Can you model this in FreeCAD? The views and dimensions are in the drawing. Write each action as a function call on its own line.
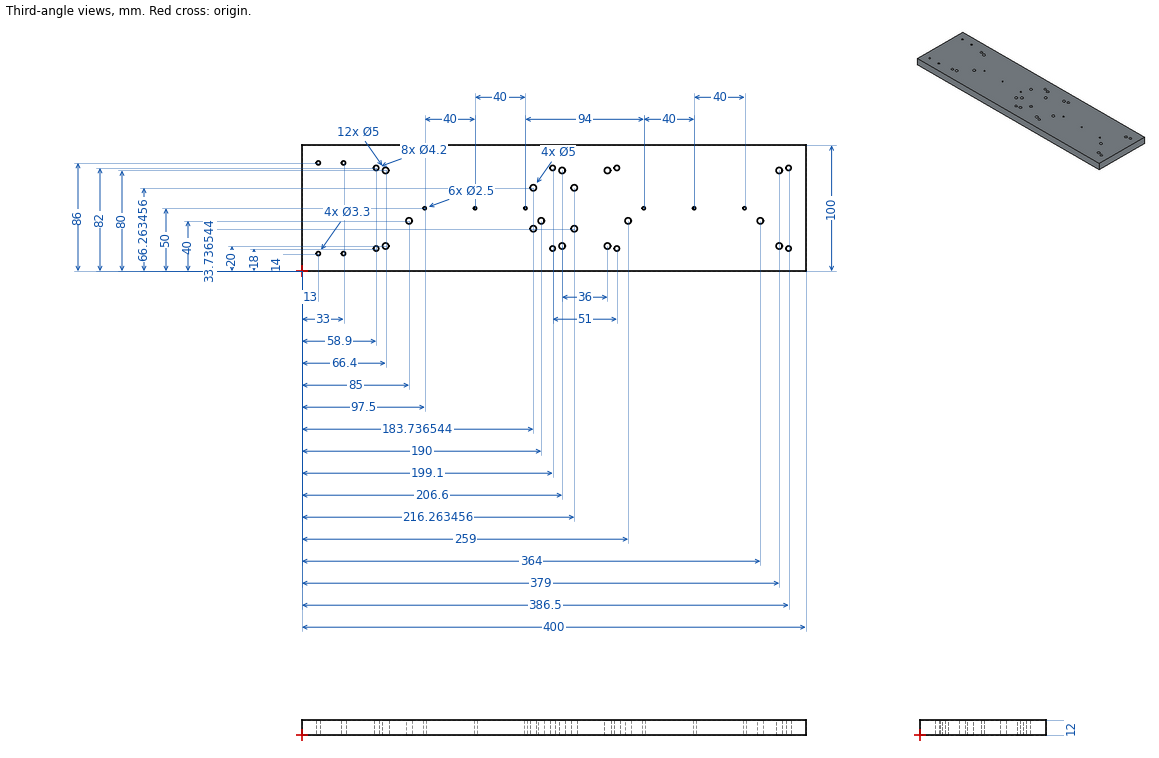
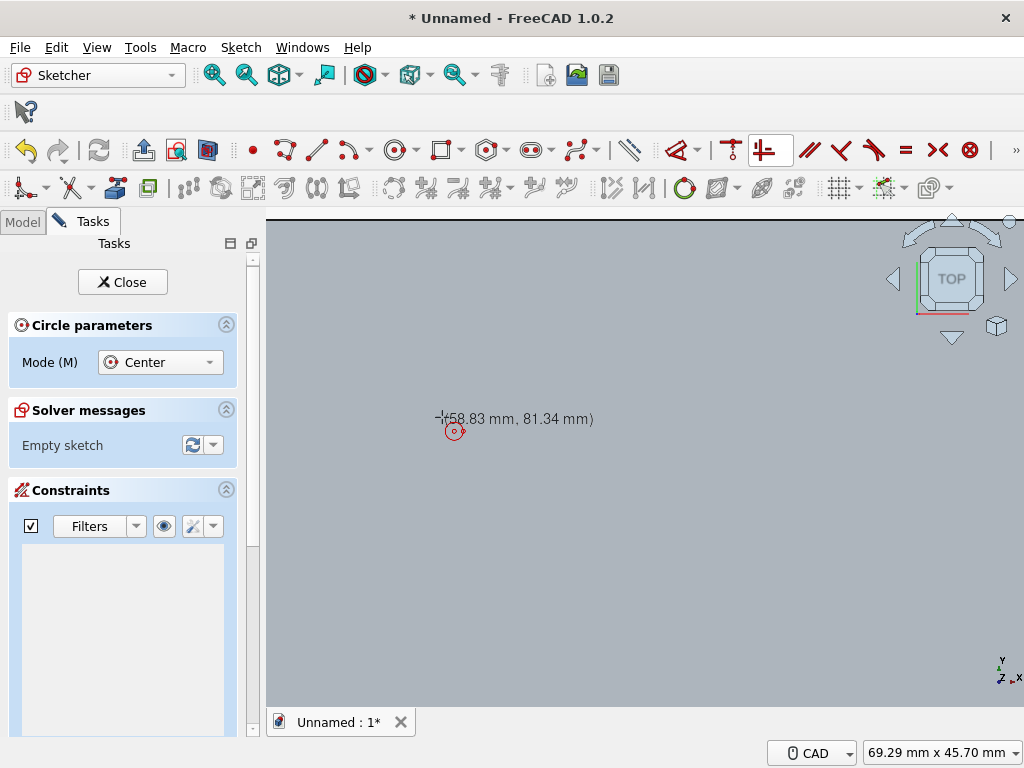
scroll(442, 417, down, 12)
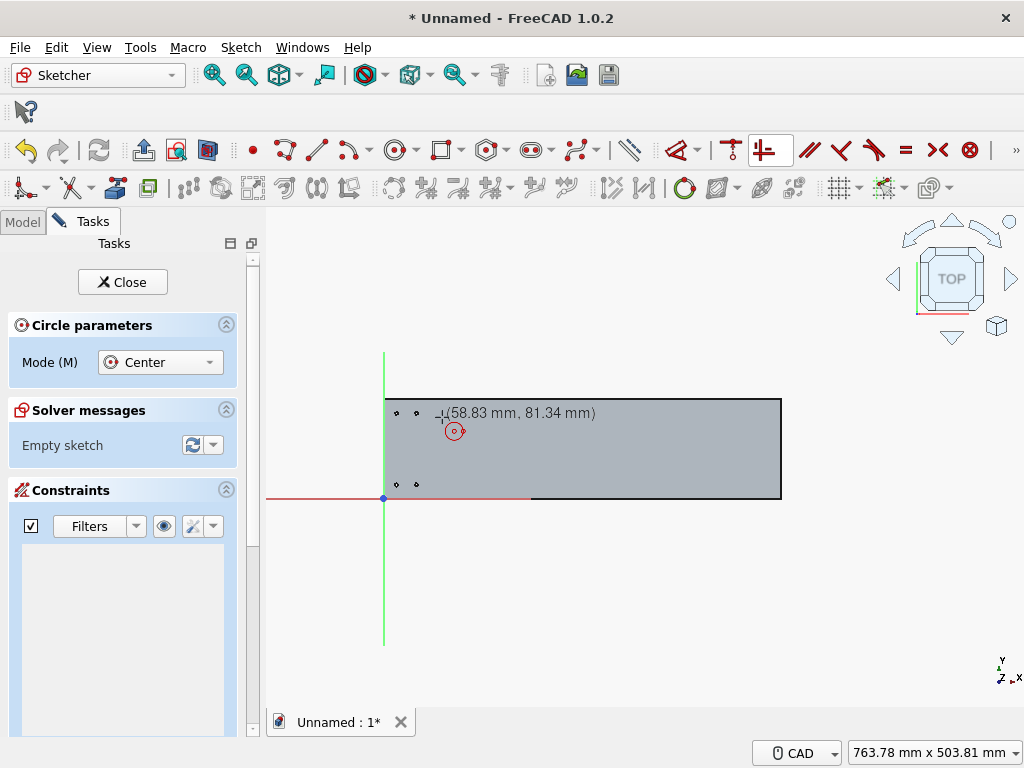
click(442, 417)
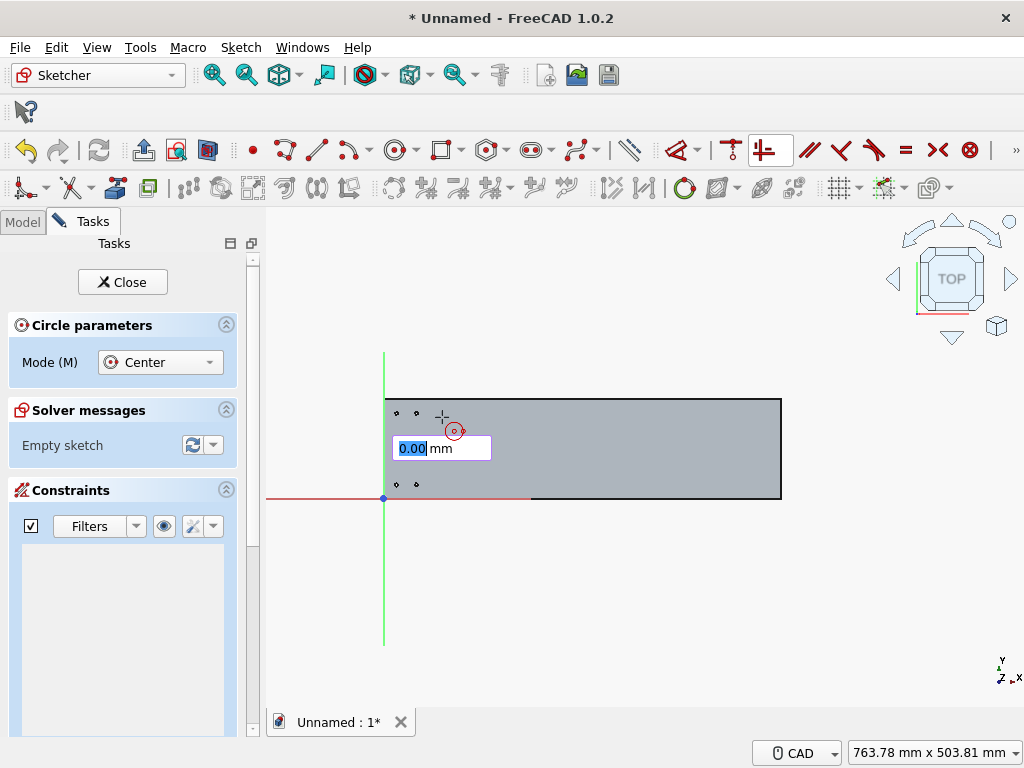
scroll(444, 416, up, 11)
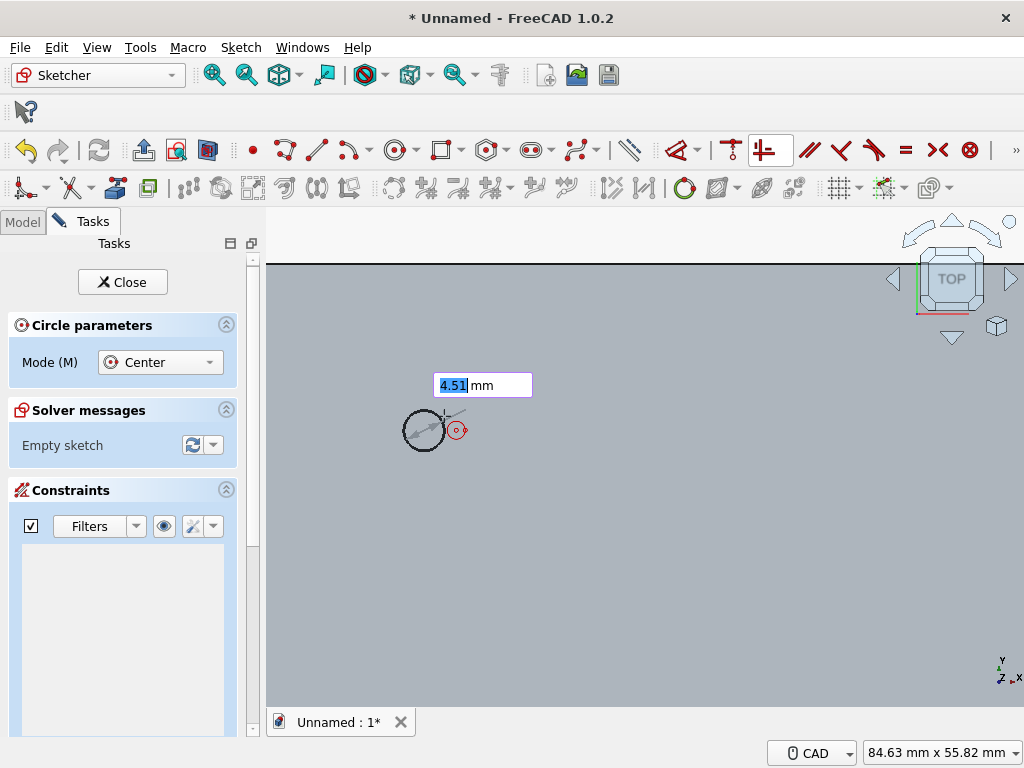
click(438, 411)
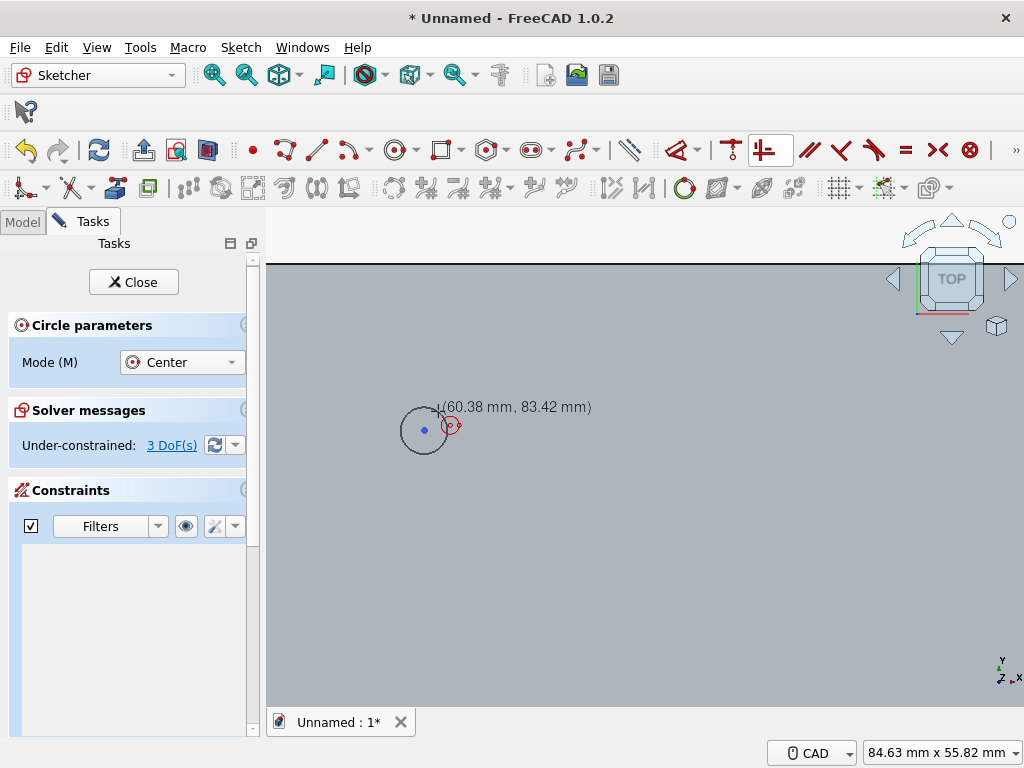
scroll(444, 416, down, 11)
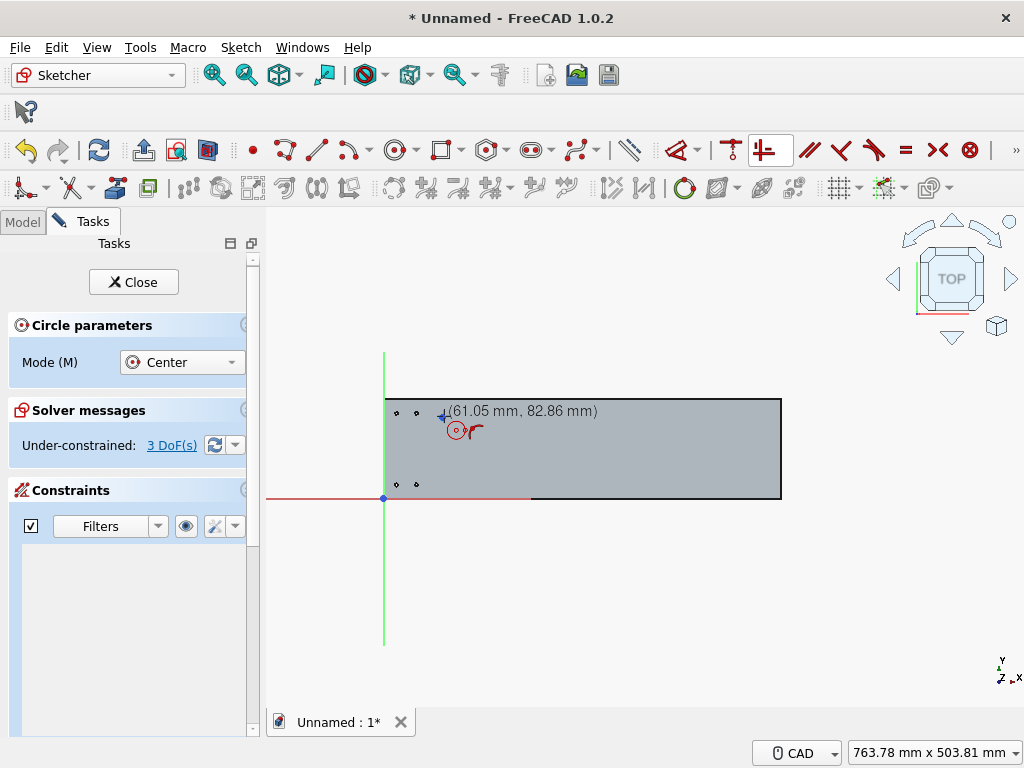
scroll(442, 481, up, 12)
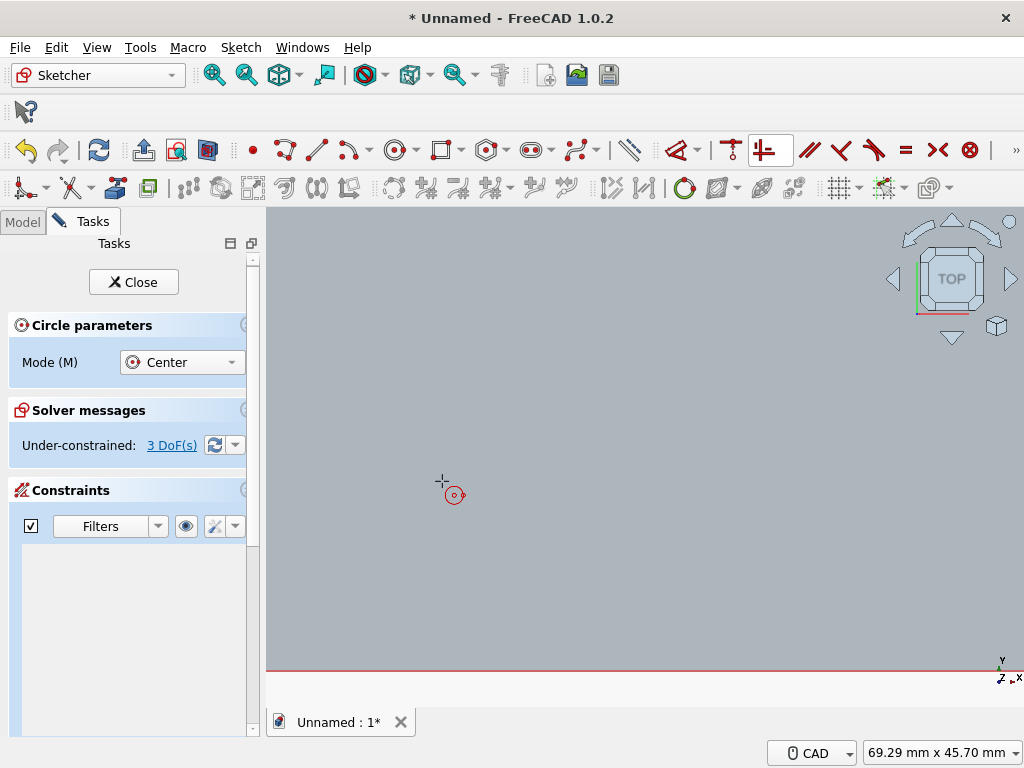
scroll(442, 482, down, 12)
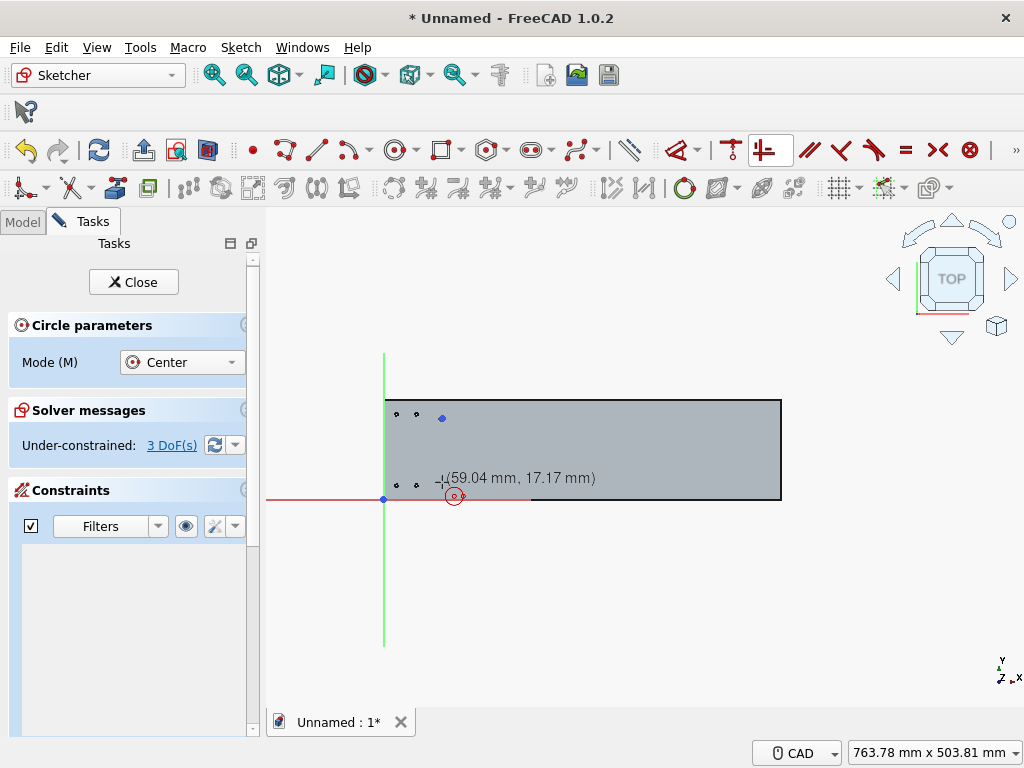
click(442, 482)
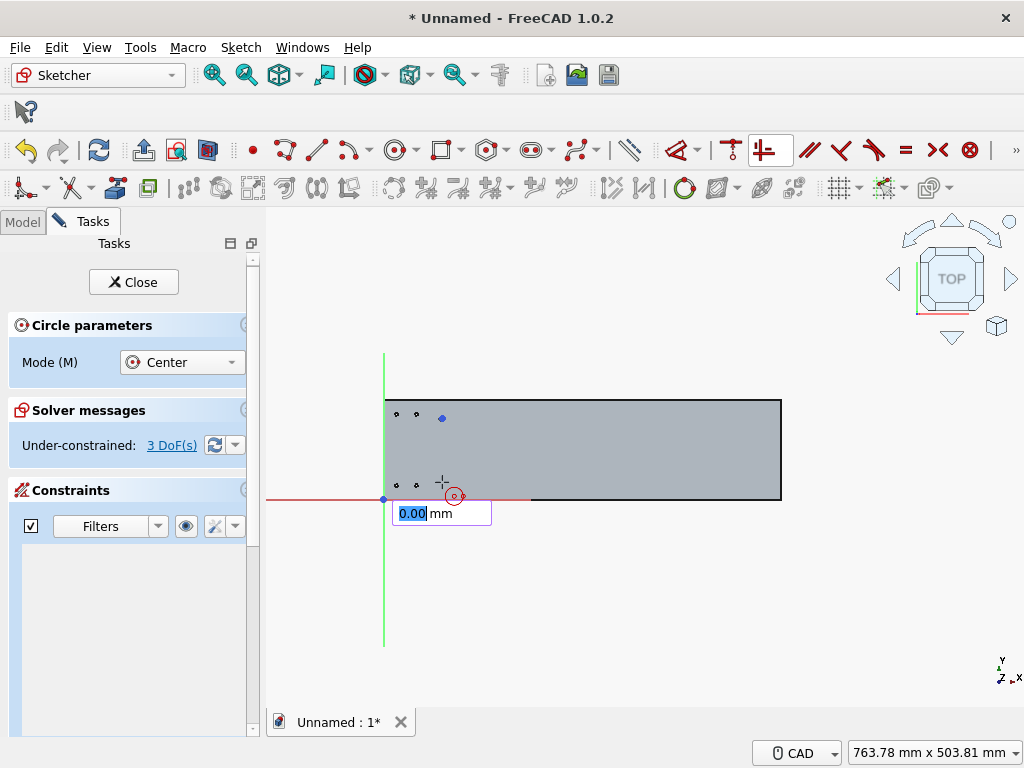
scroll(444, 480, up, 11)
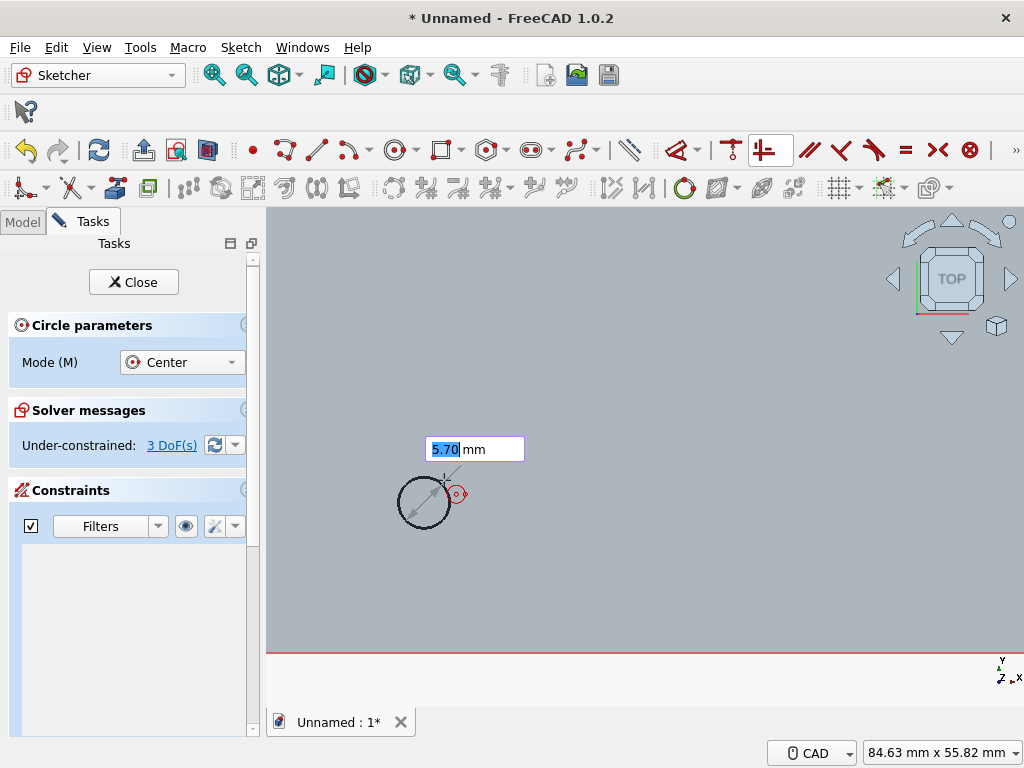
click(438, 478)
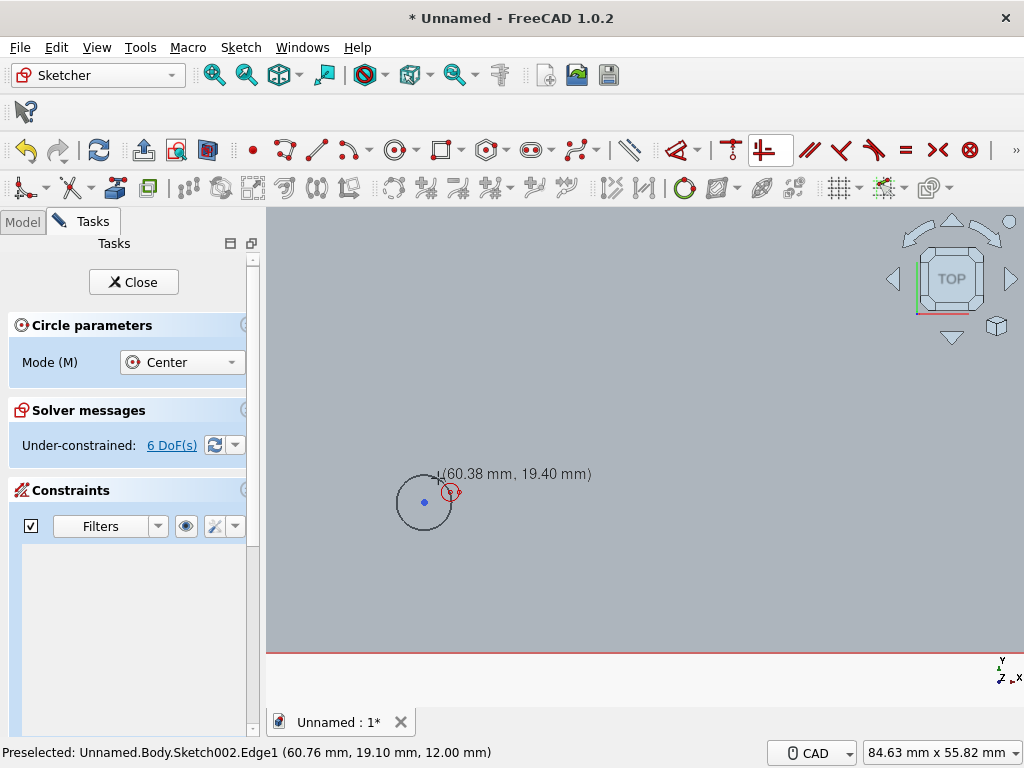
scroll(444, 480, down, 11)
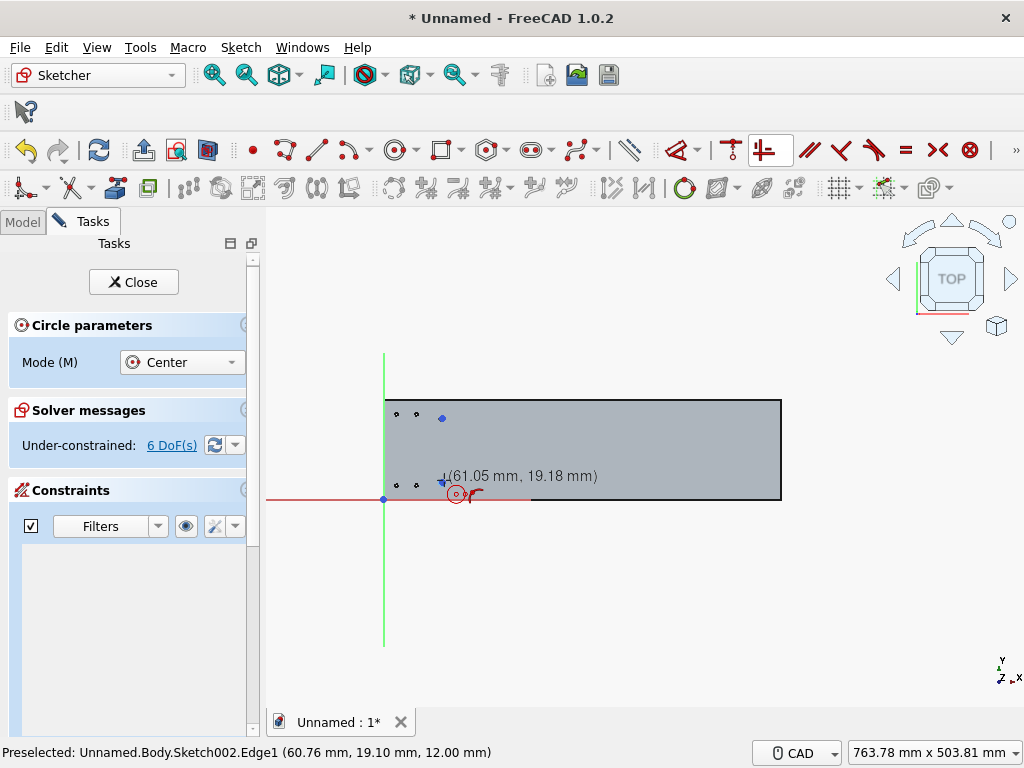
scroll(581, 418, up, 12)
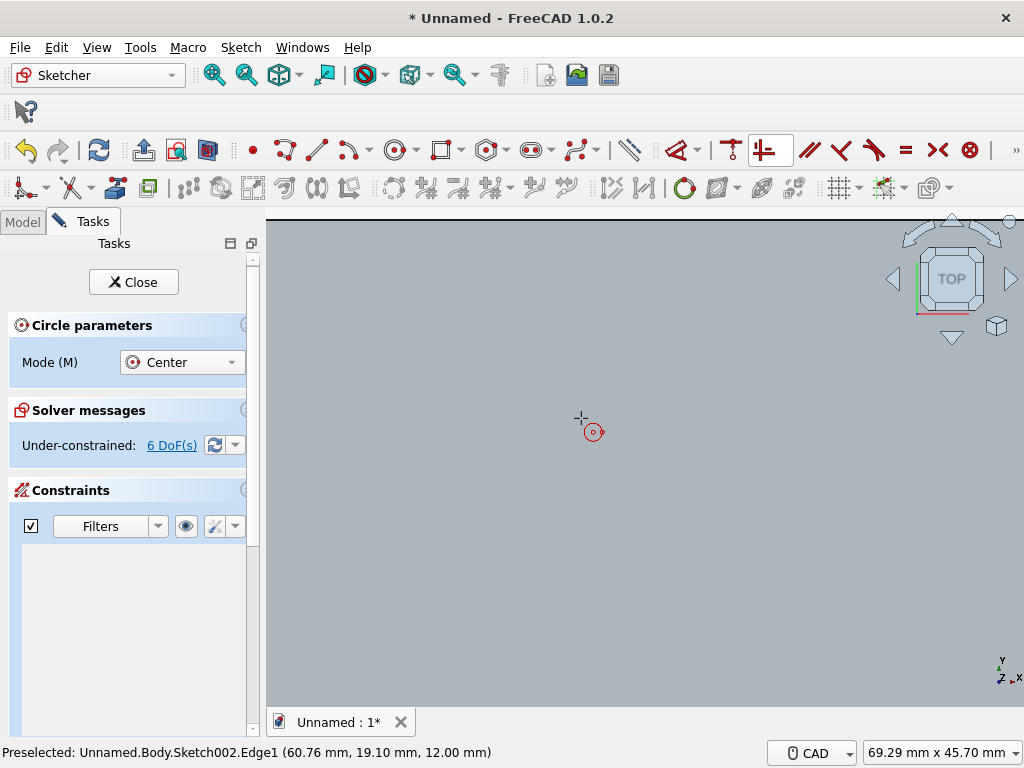
scroll(581, 417, down, 12)